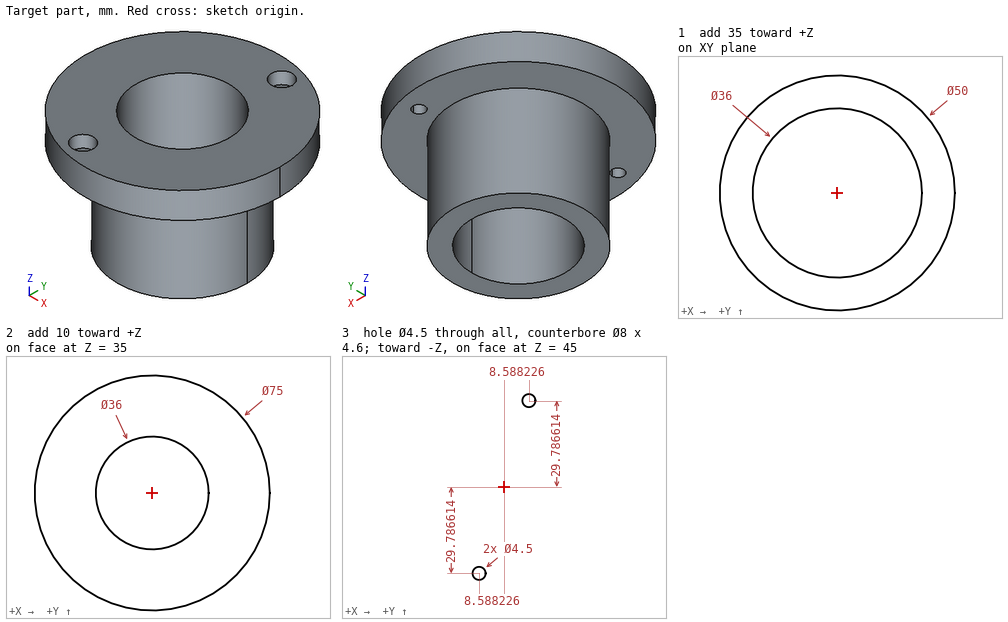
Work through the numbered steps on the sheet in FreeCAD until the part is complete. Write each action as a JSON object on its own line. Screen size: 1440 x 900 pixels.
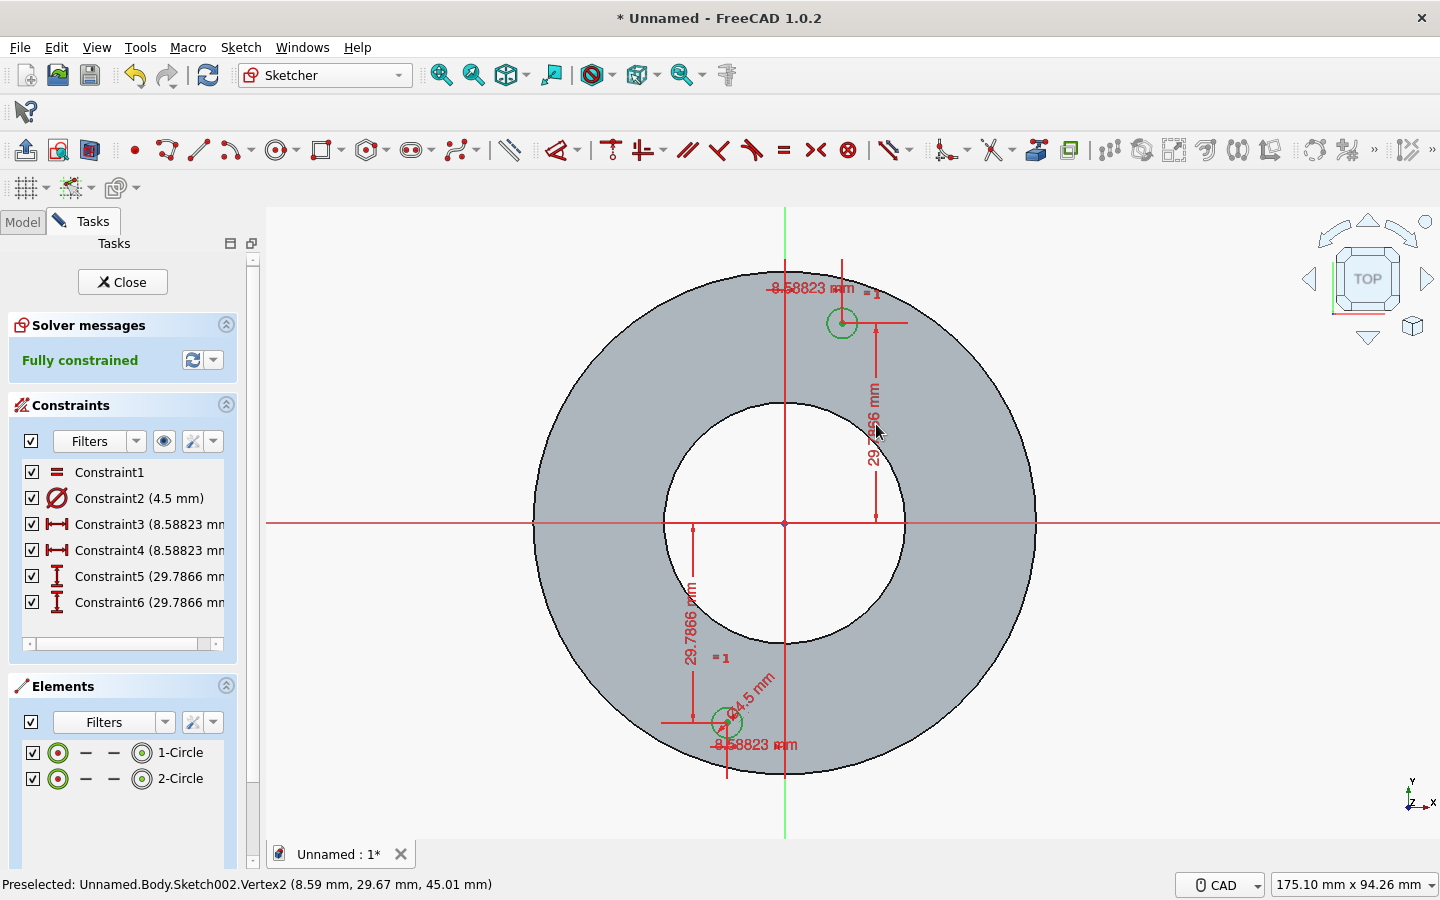
{"action": "left_click", "coordinate": [123, 282]}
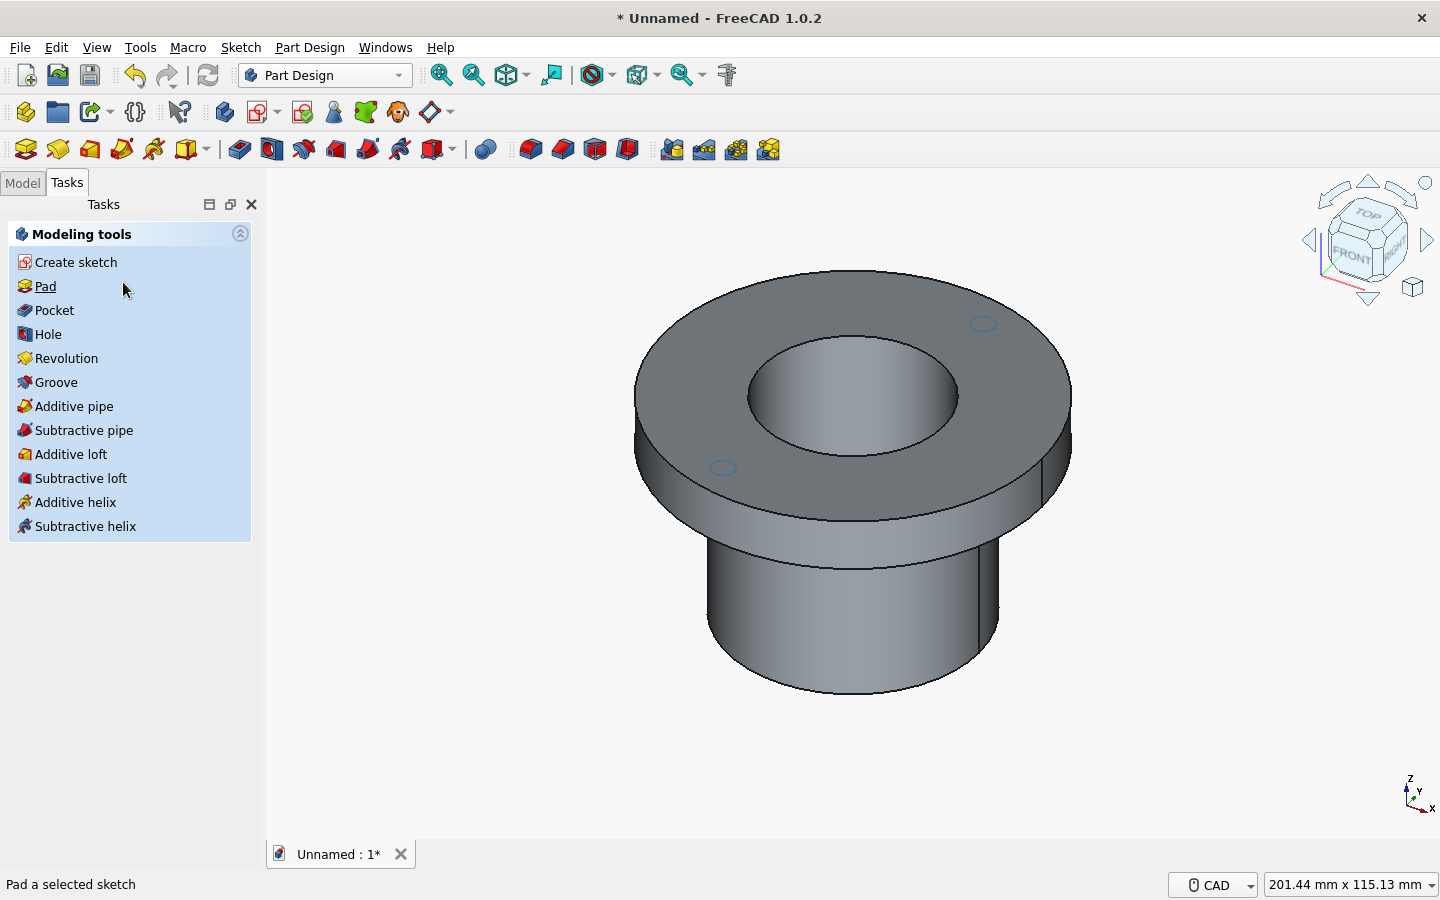
{"action": "left_click", "coordinate": [272, 150]}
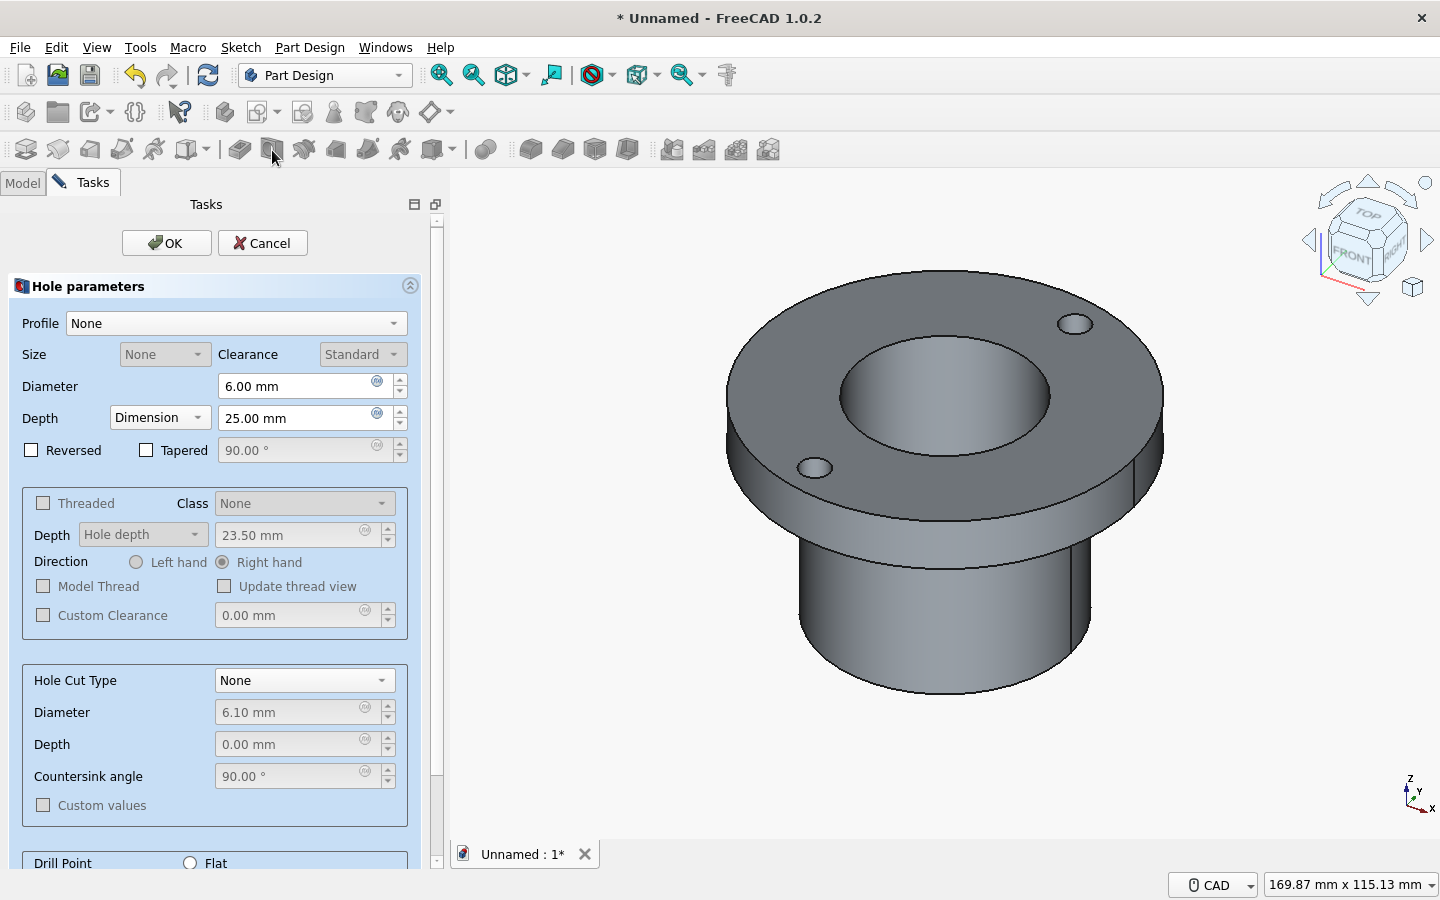
{"action": "triple_click", "coordinate": [305, 386]}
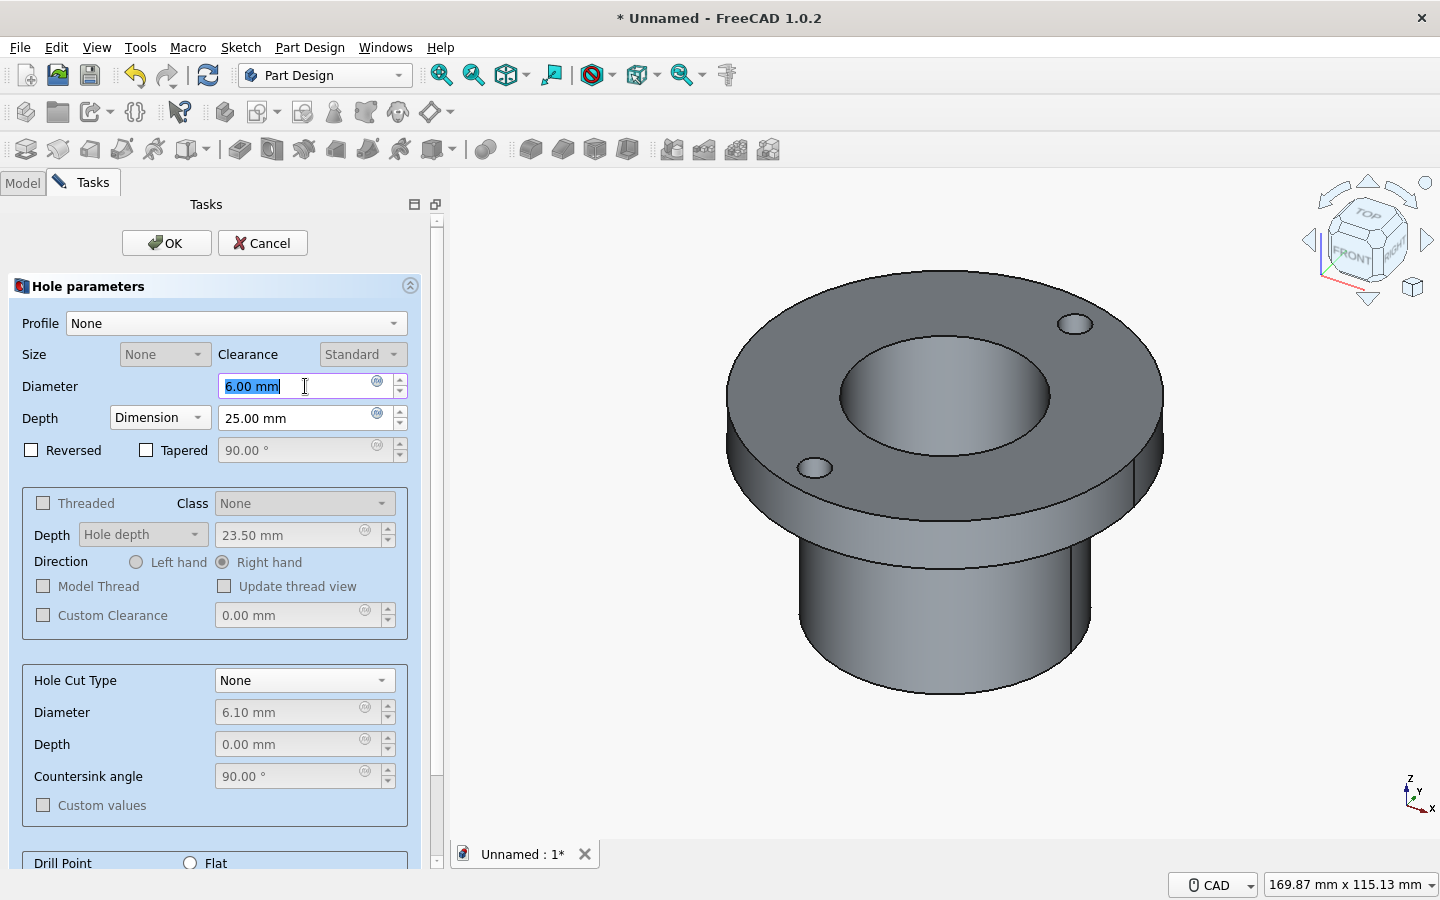
{"action": "type", "text": "4.5"}
{"action": "key", "text": "Tab"}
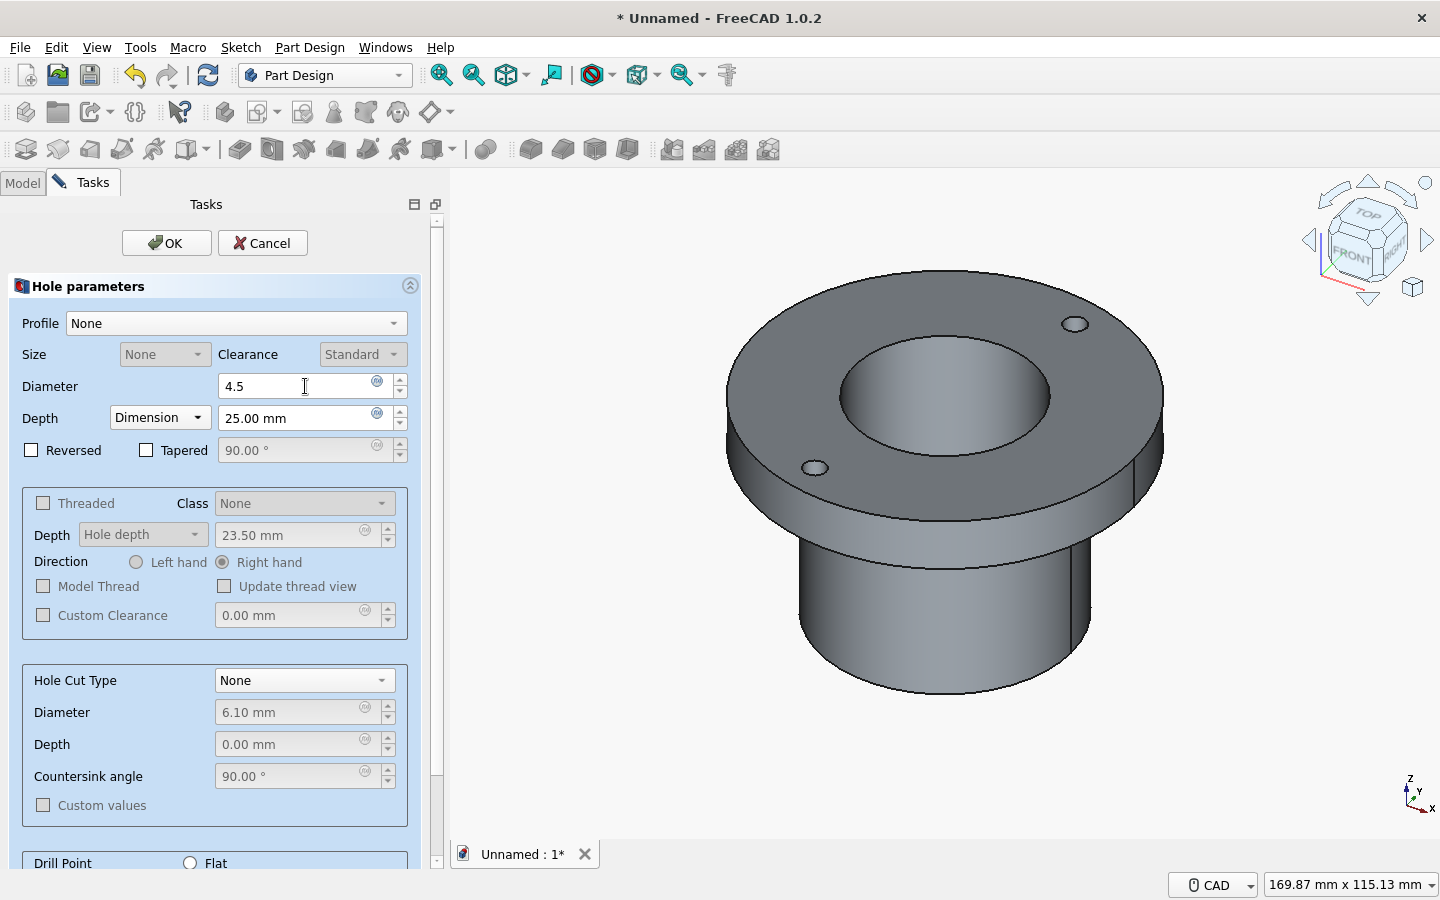
{"action": "left_click", "coordinate": [161, 418]}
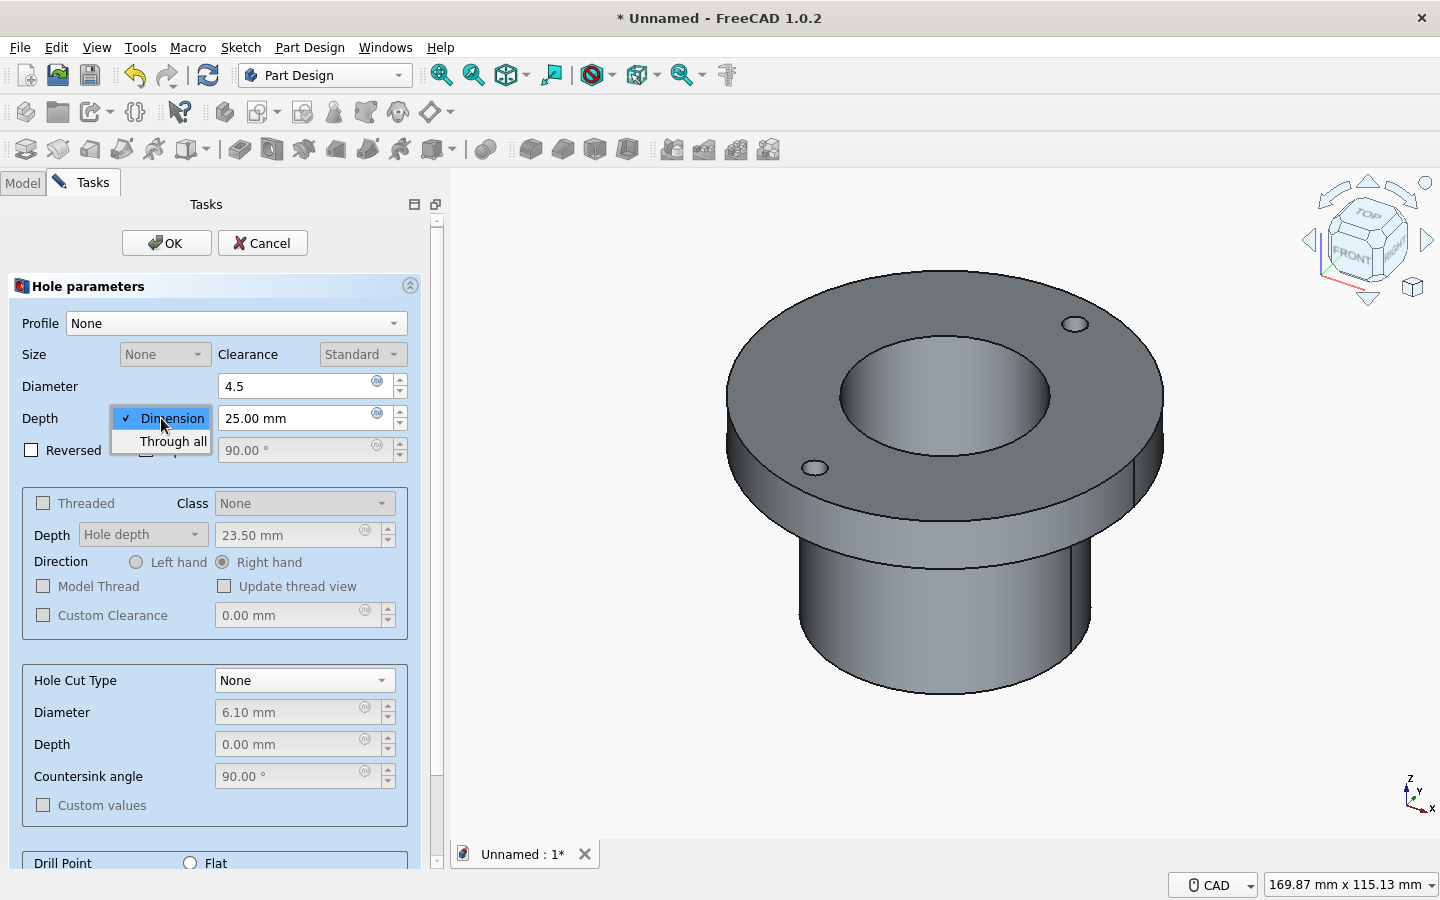
{"action": "left_click", "coordinate": [160, 442]}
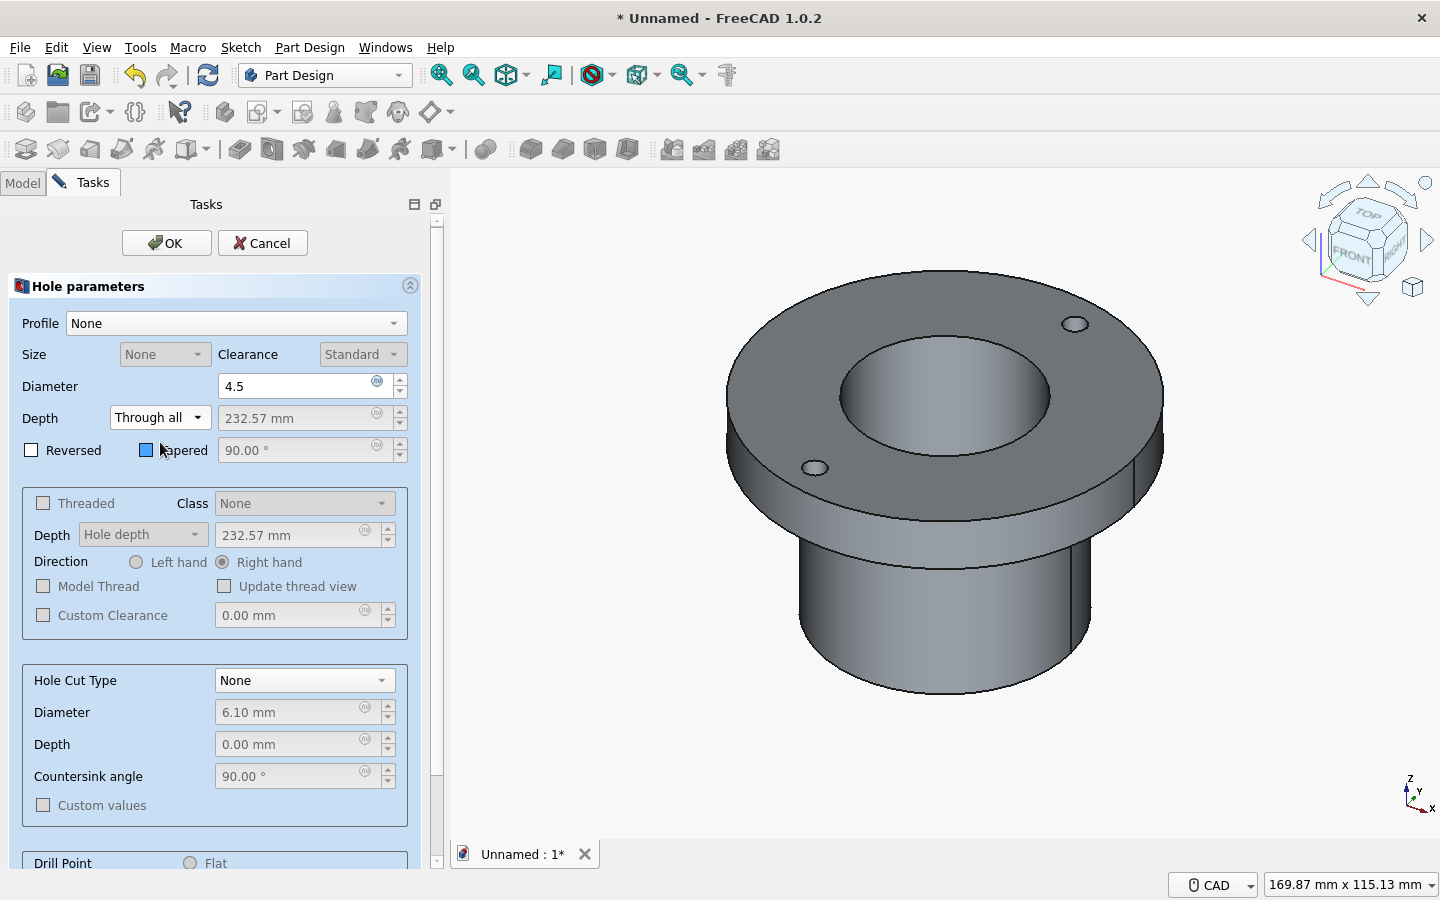
{"action": "left_click", "coordinate": [306, 680]}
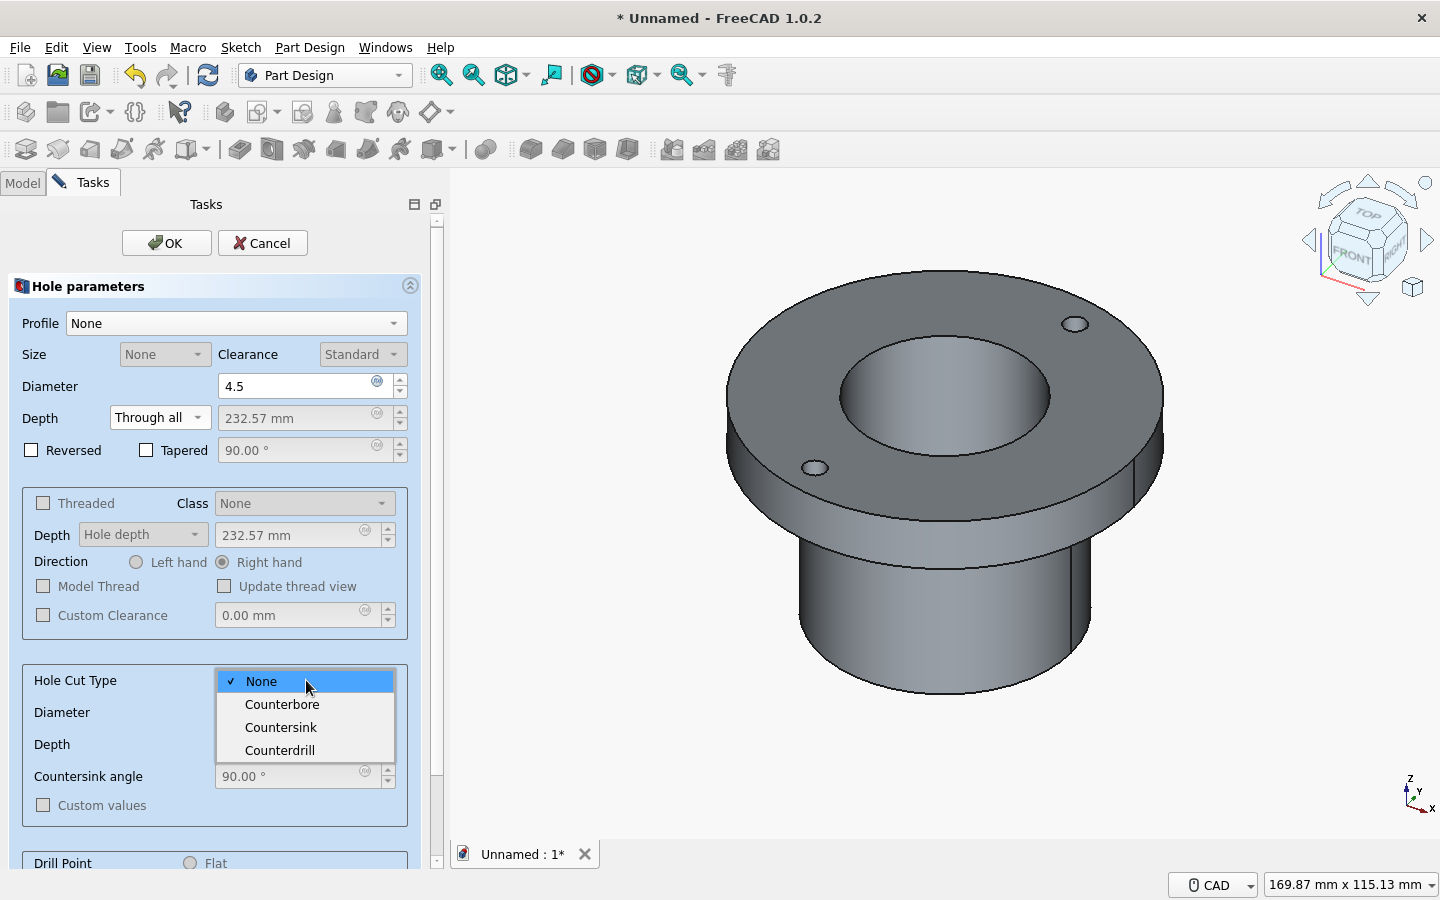
{"action": "left_click", "coordinate": [304, 704]}